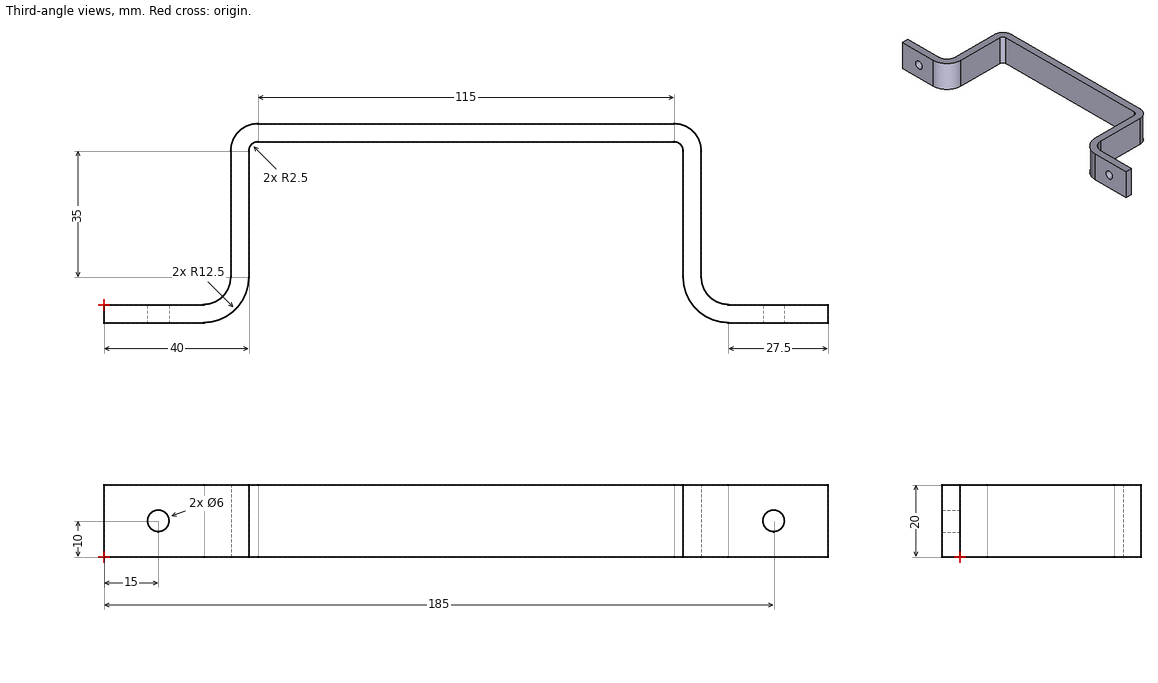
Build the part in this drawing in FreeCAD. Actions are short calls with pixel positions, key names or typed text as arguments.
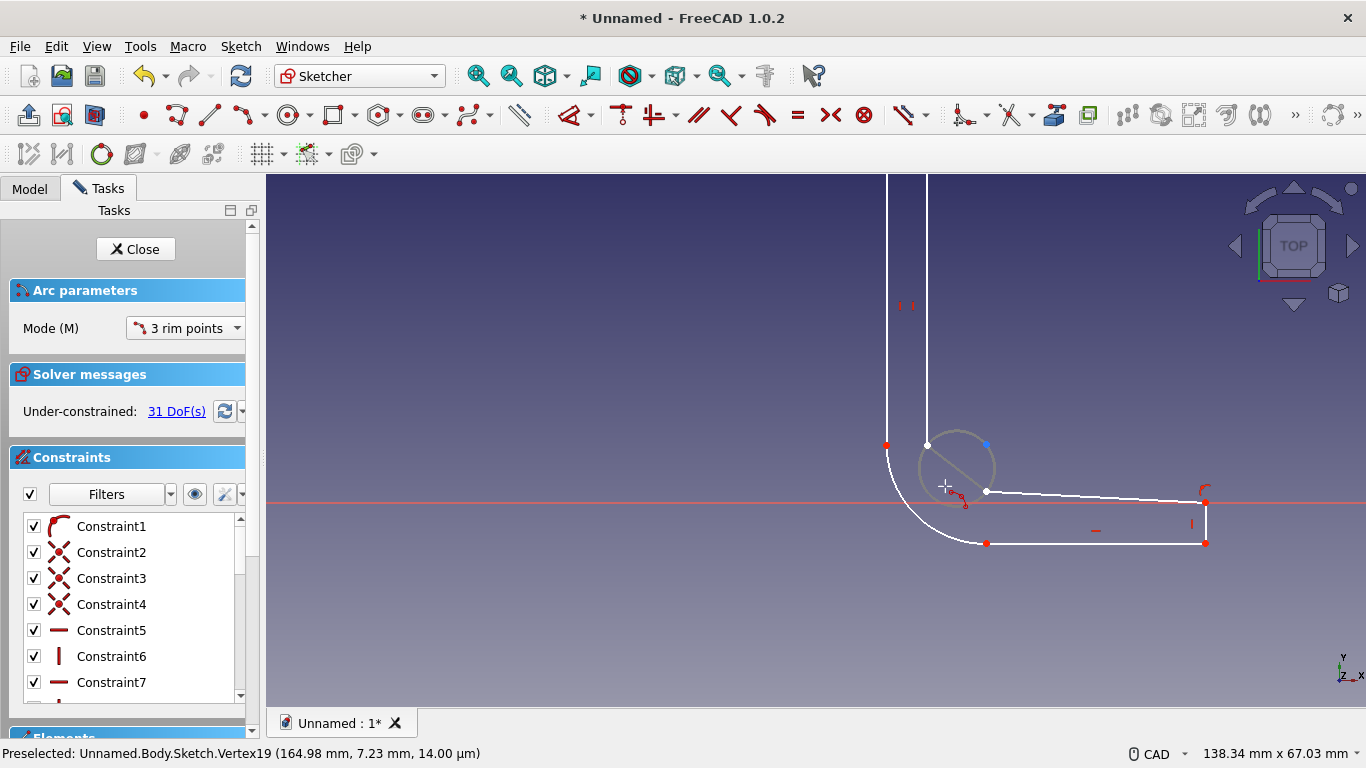
click(945, 485)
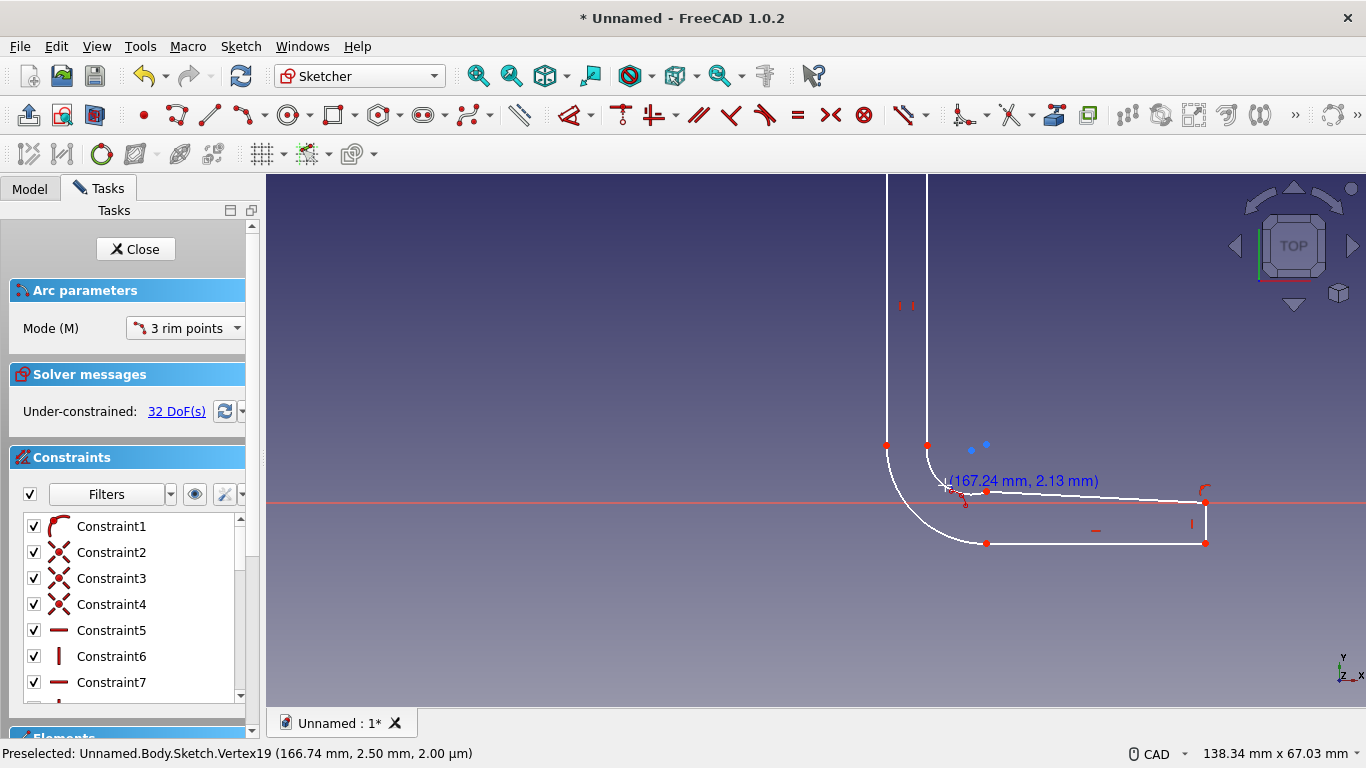
scroll(944, 508, down, 5)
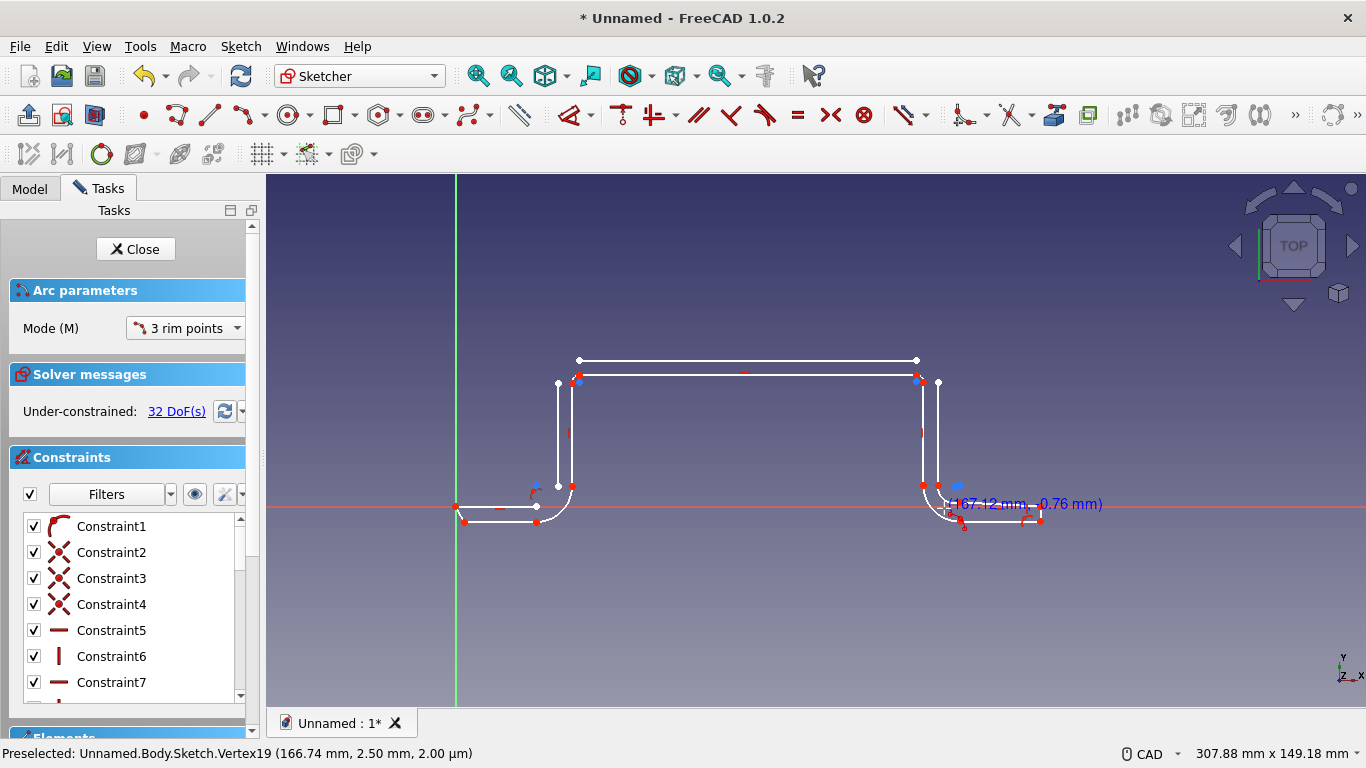
click(938, 383)
click(916, 361)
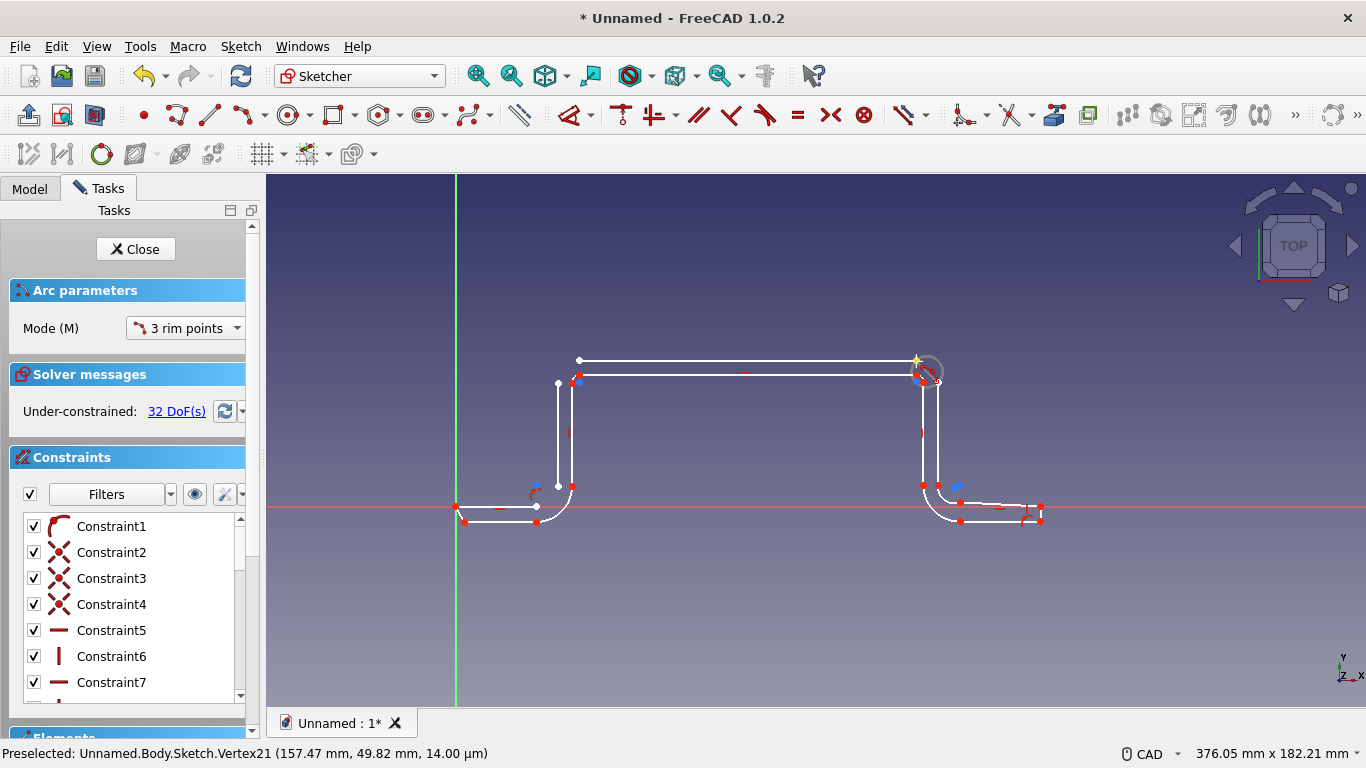
scroll(932, 367, up, 5)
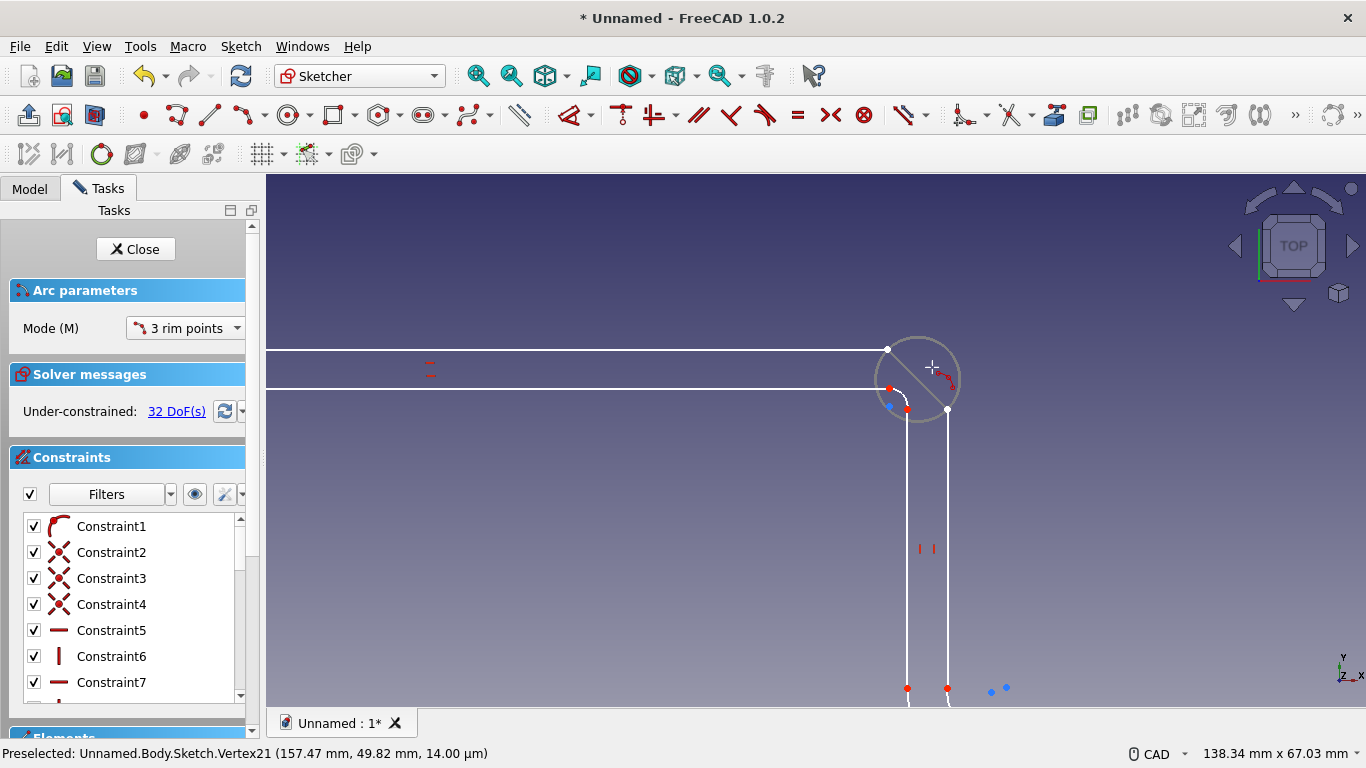
click(930, 366)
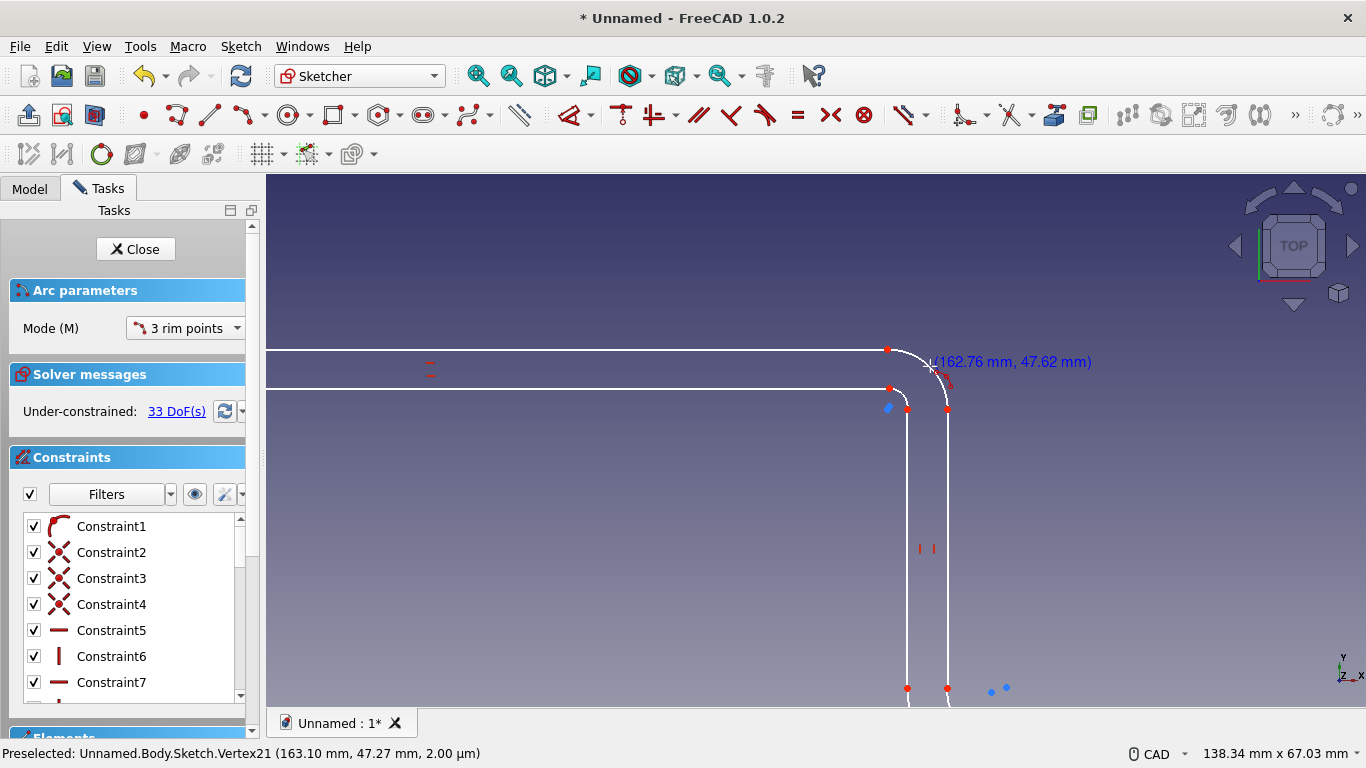
scroll(932, 367, down, 5)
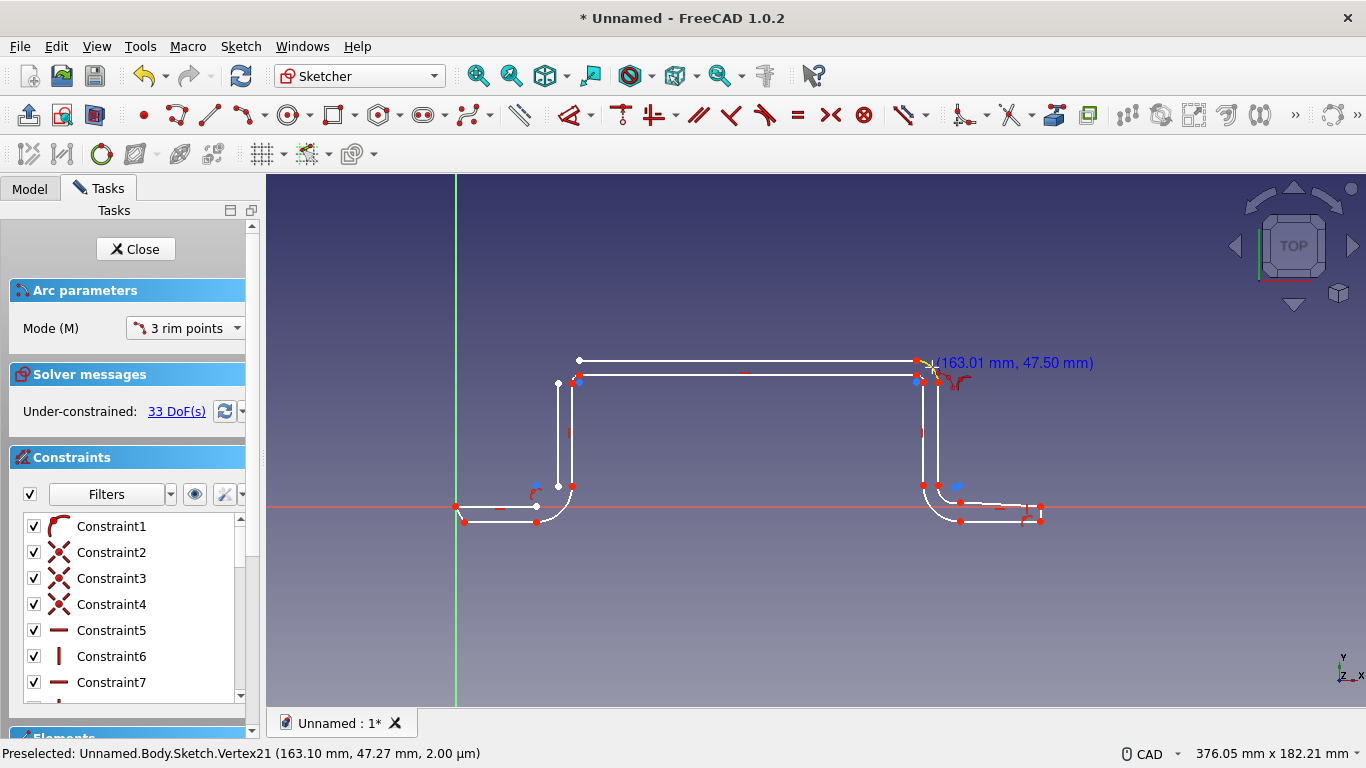
click(580, 361)
click(558, 383)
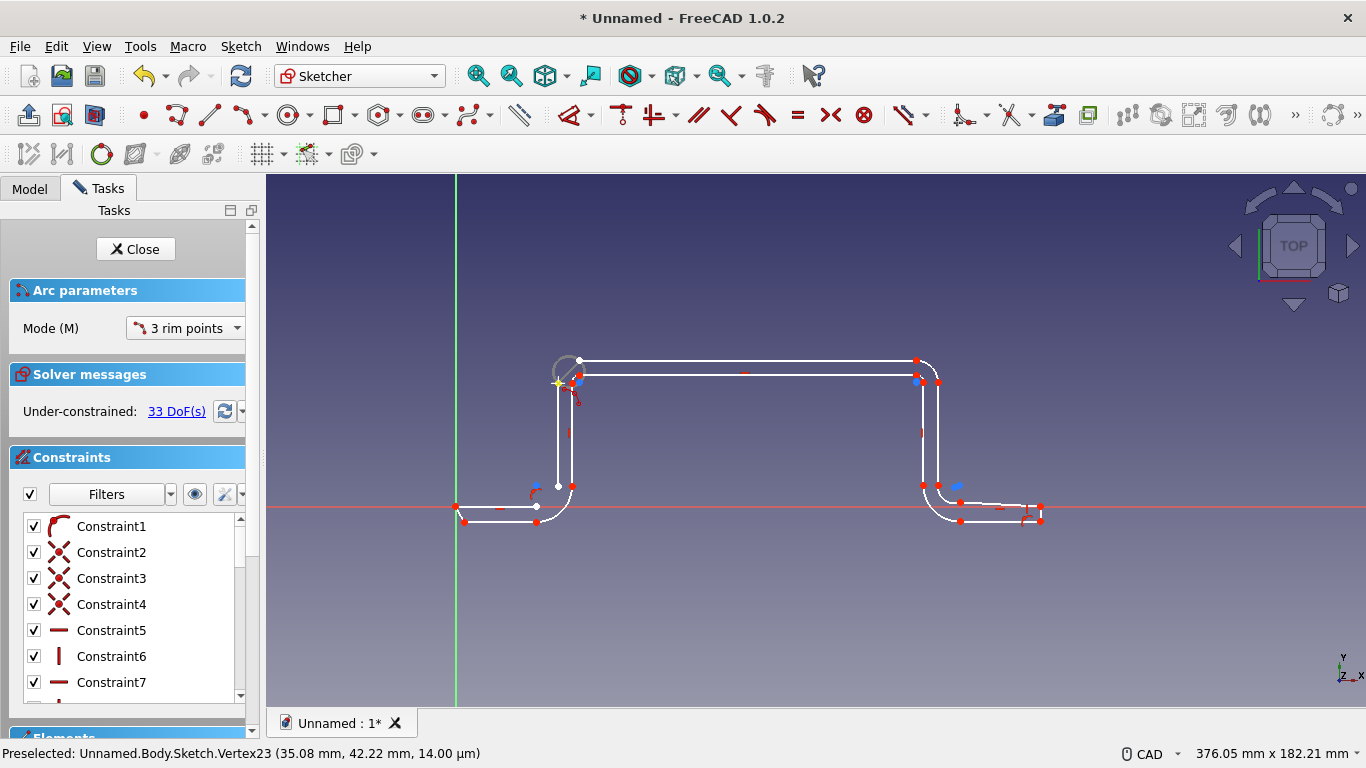
scroll(564, 367, up, 5)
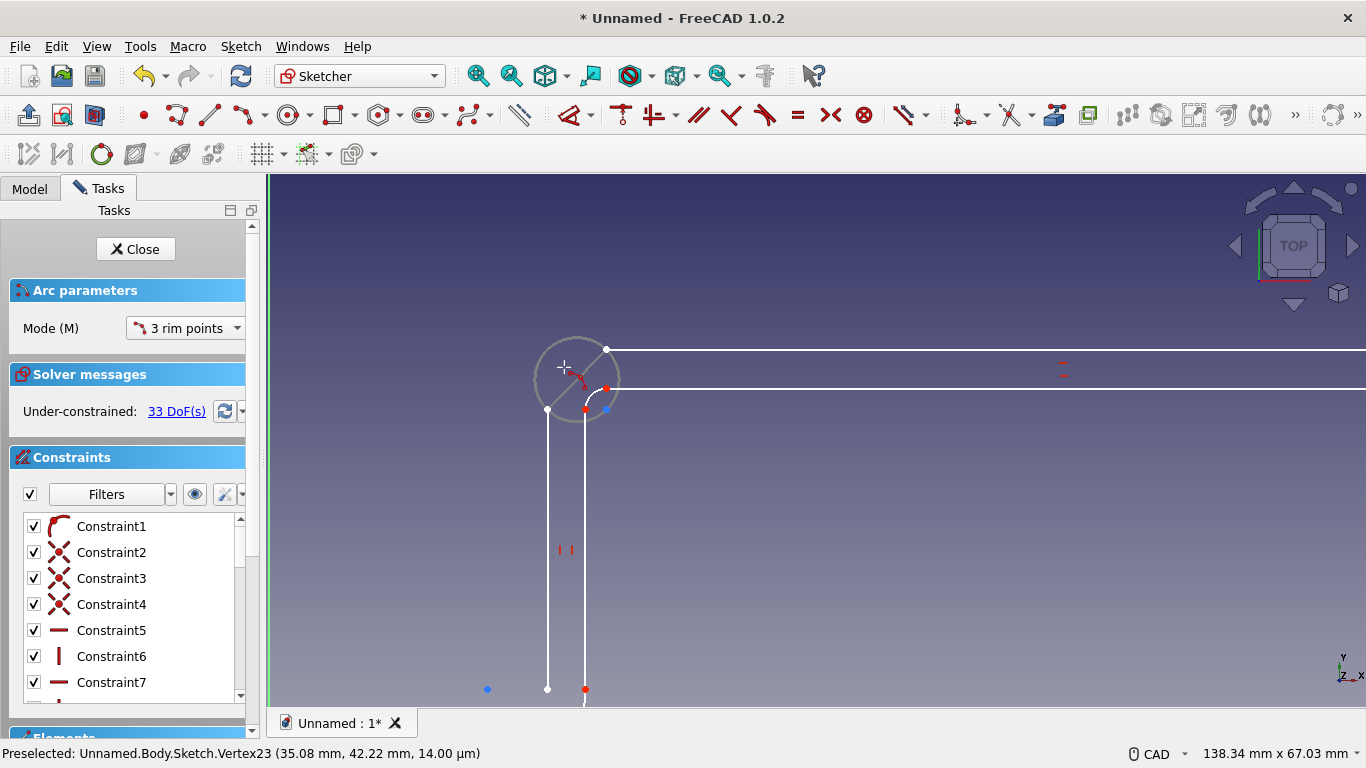
click(564, 366)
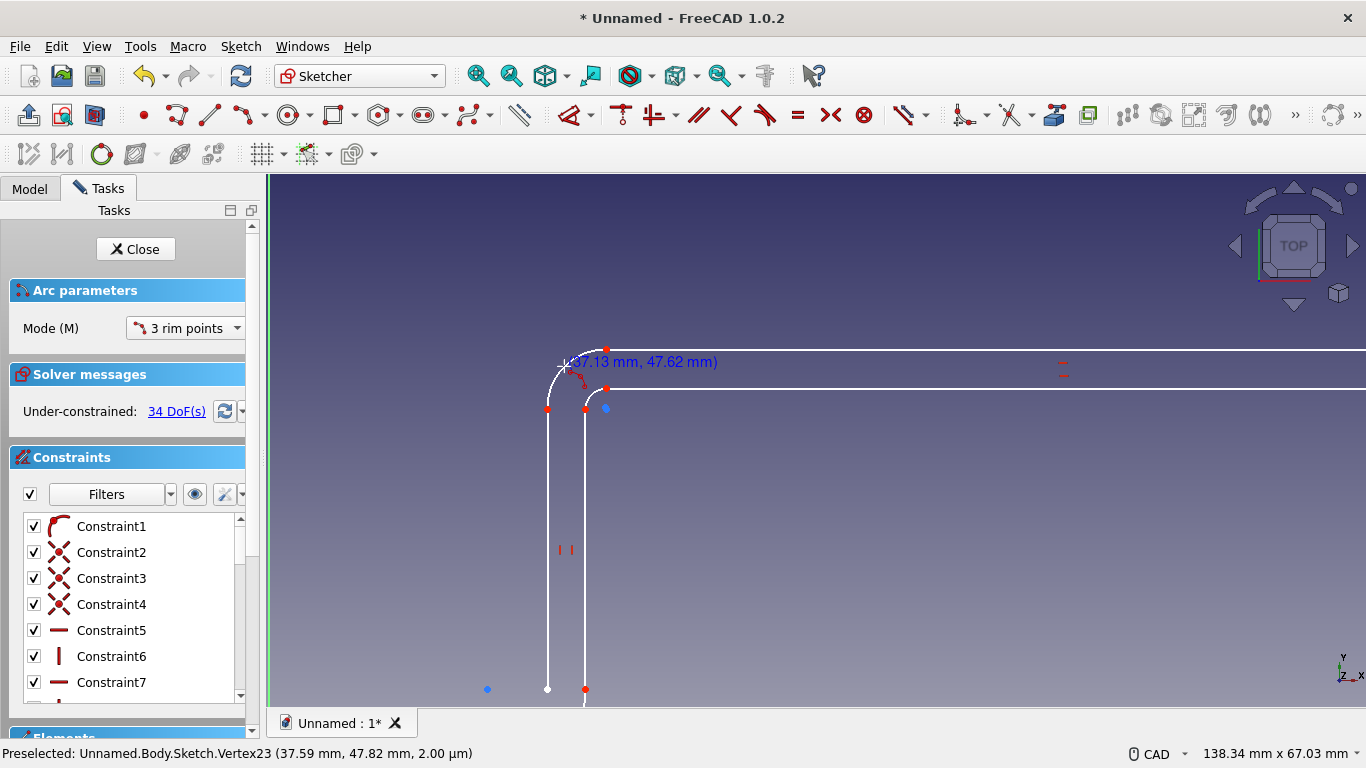
scroll(563, 367, down, 5)